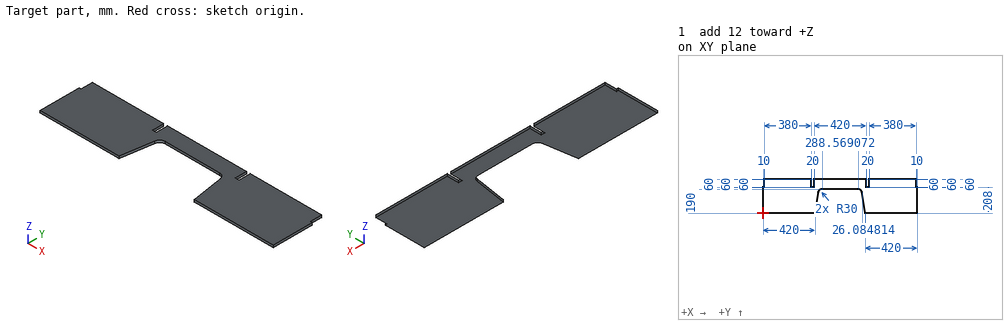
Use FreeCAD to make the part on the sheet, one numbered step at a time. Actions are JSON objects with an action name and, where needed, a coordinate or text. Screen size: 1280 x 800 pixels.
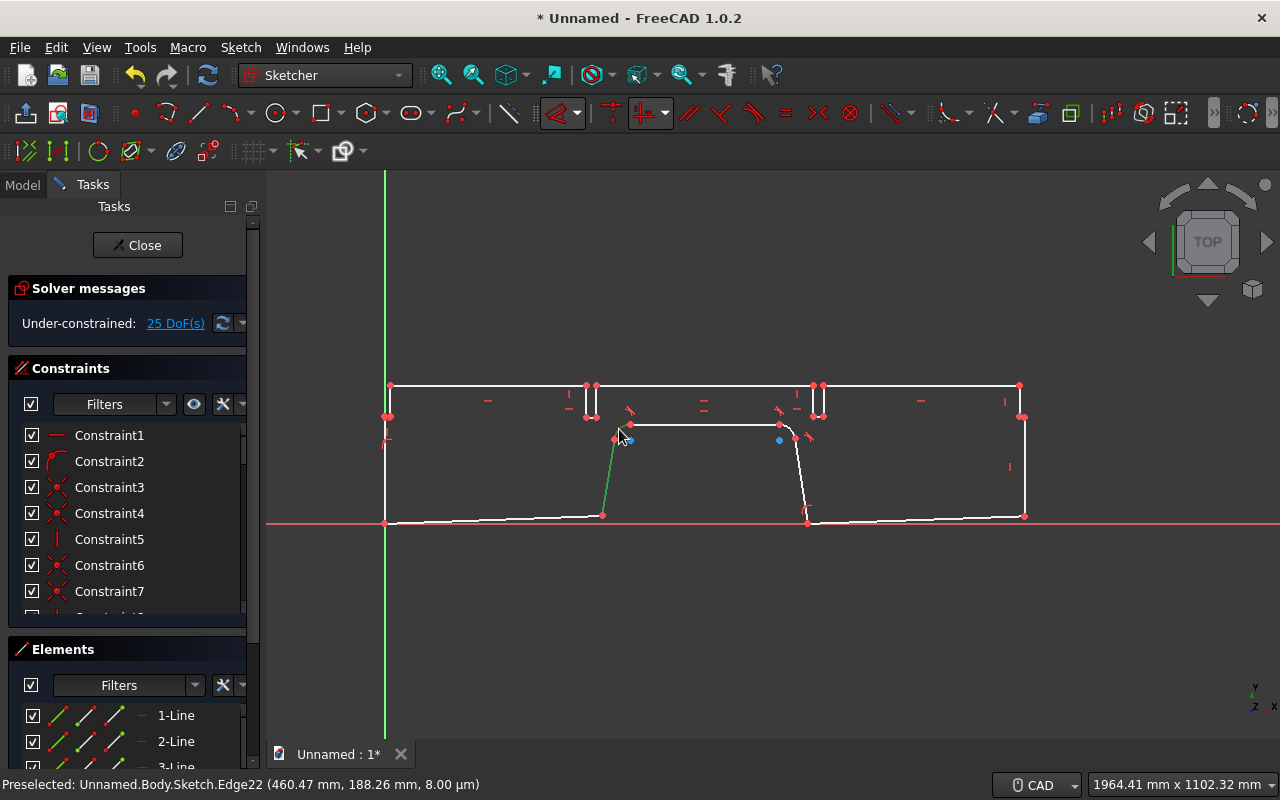
{"action": "key", "text": "t"}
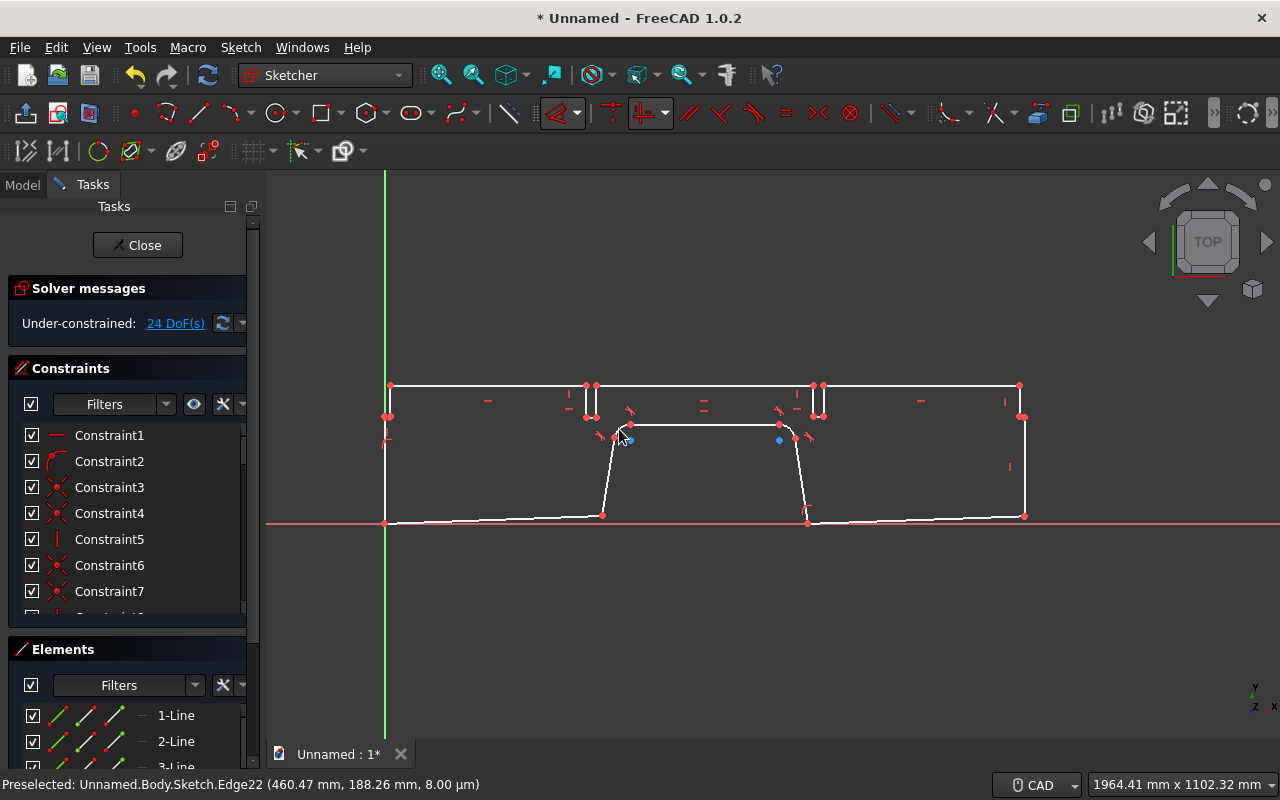
{"action": "left_click", "coordinate": [873, 522]}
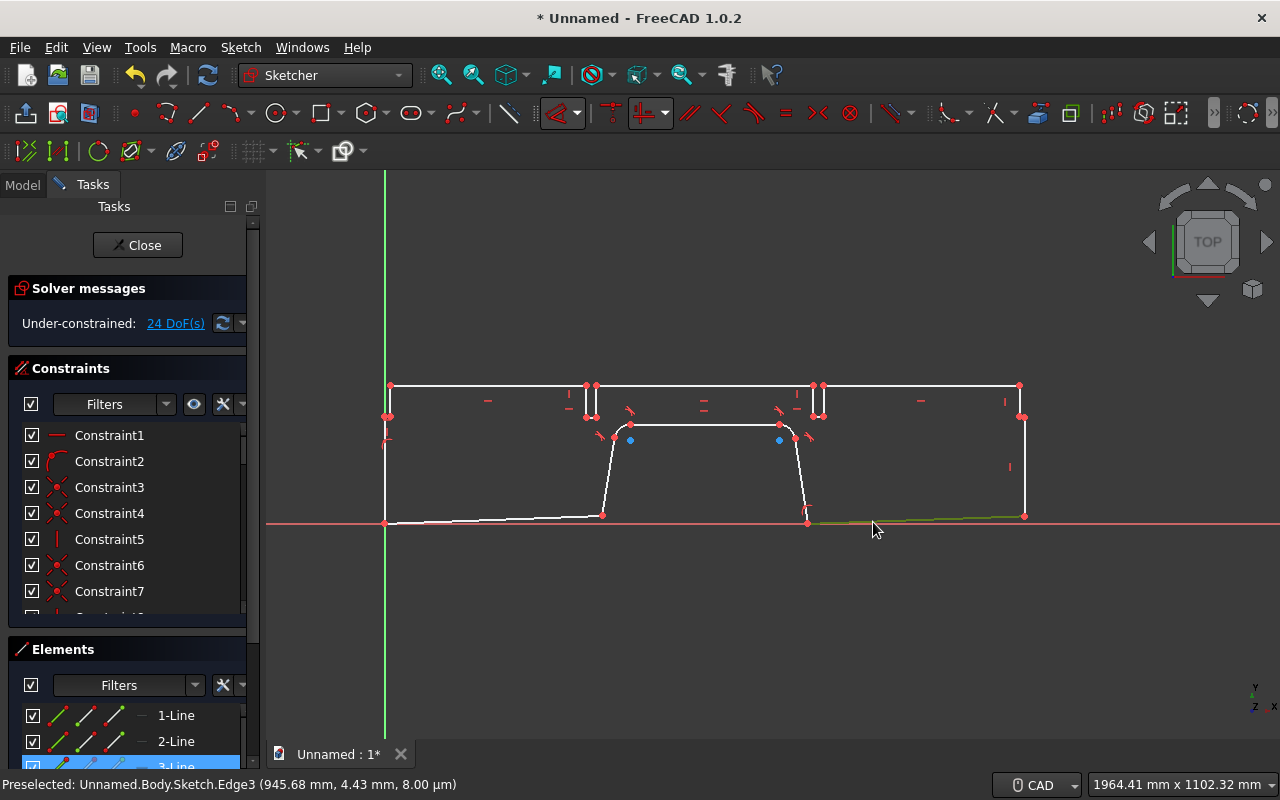
{"action": "key", "text": "h"}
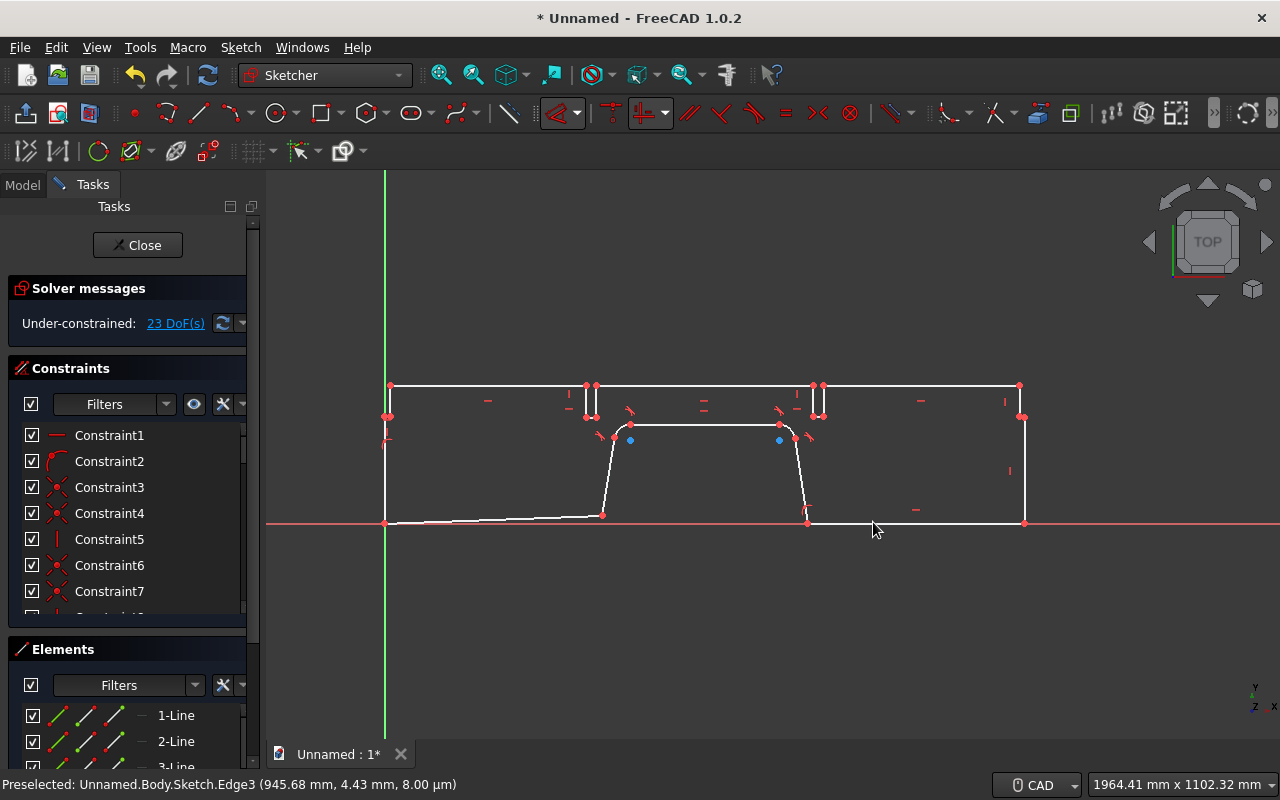
{"action": "scroll", "coordinate": [1022, 417], "scroll_direction": "up", "scroll_amount": 9}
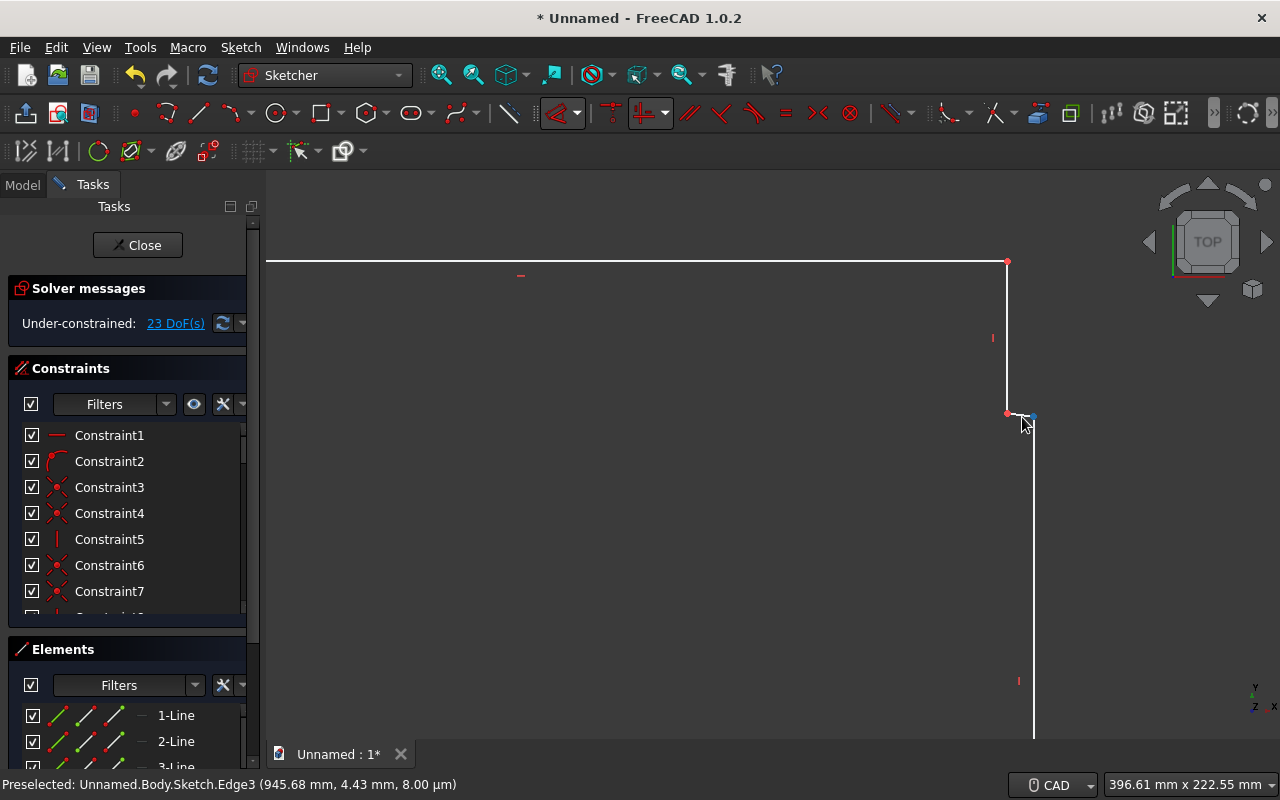
{"action": "left_click", "coordinate": [1020, 415]}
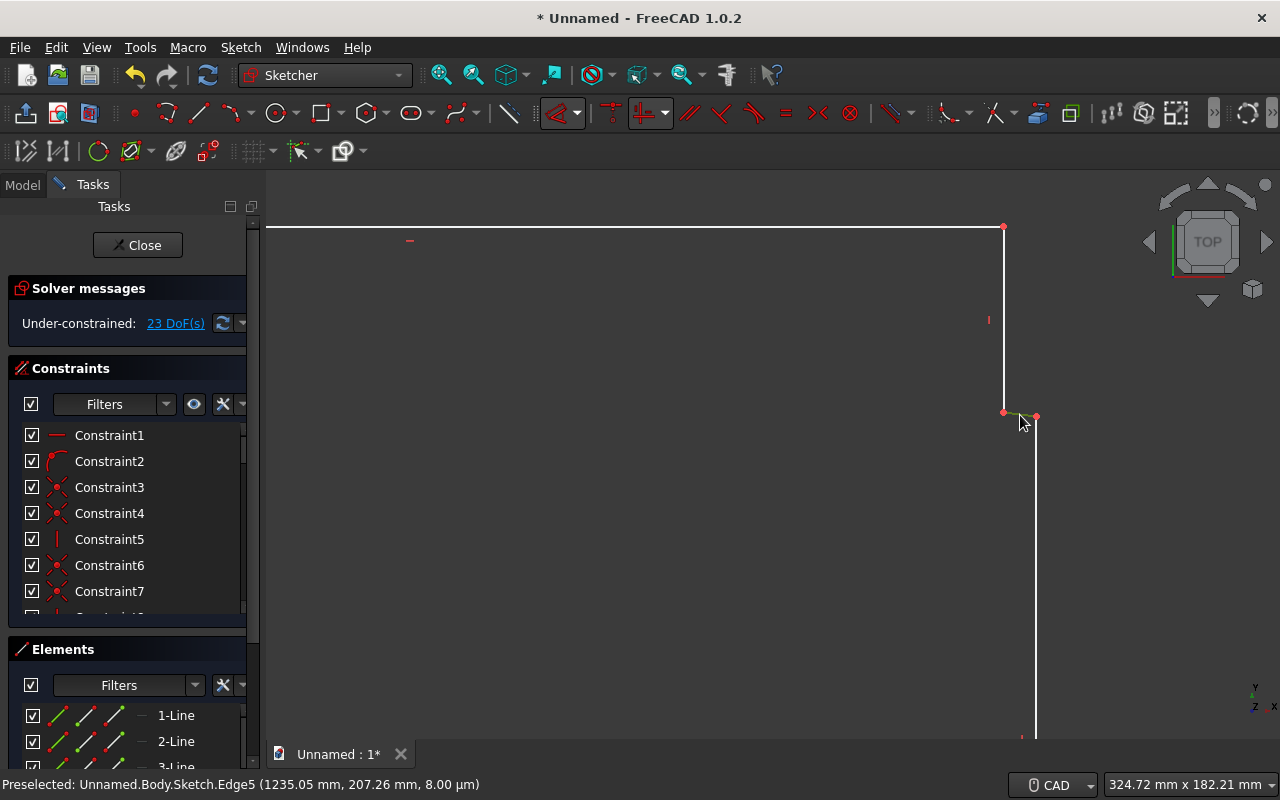
{"action": "key", "text": "h"}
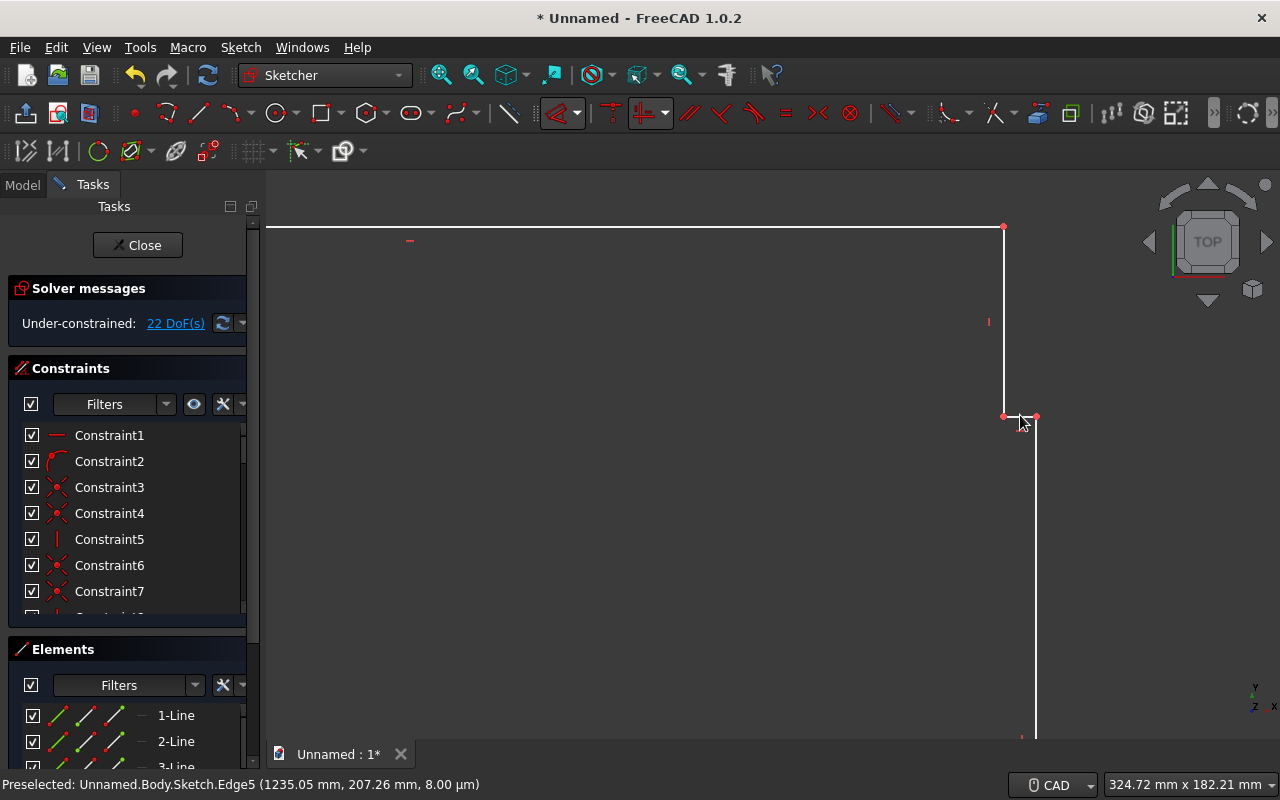
{"action": "scroll", "coordinate": [1022, 417], "scroll_direction": "down", "scroll_amount": 9}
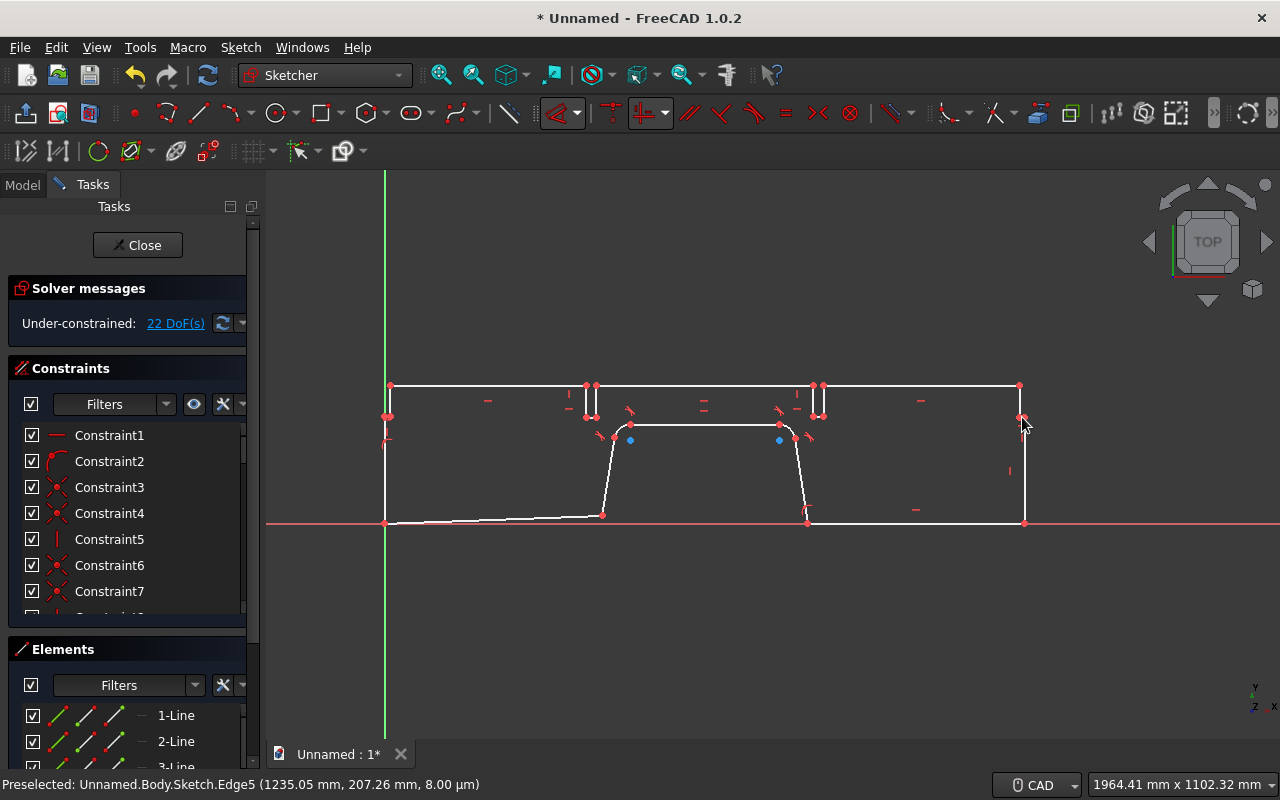
{"action": "scroll", "coordinate": [450, 522], "scroll_direction": "up", "scroll_amount": 9}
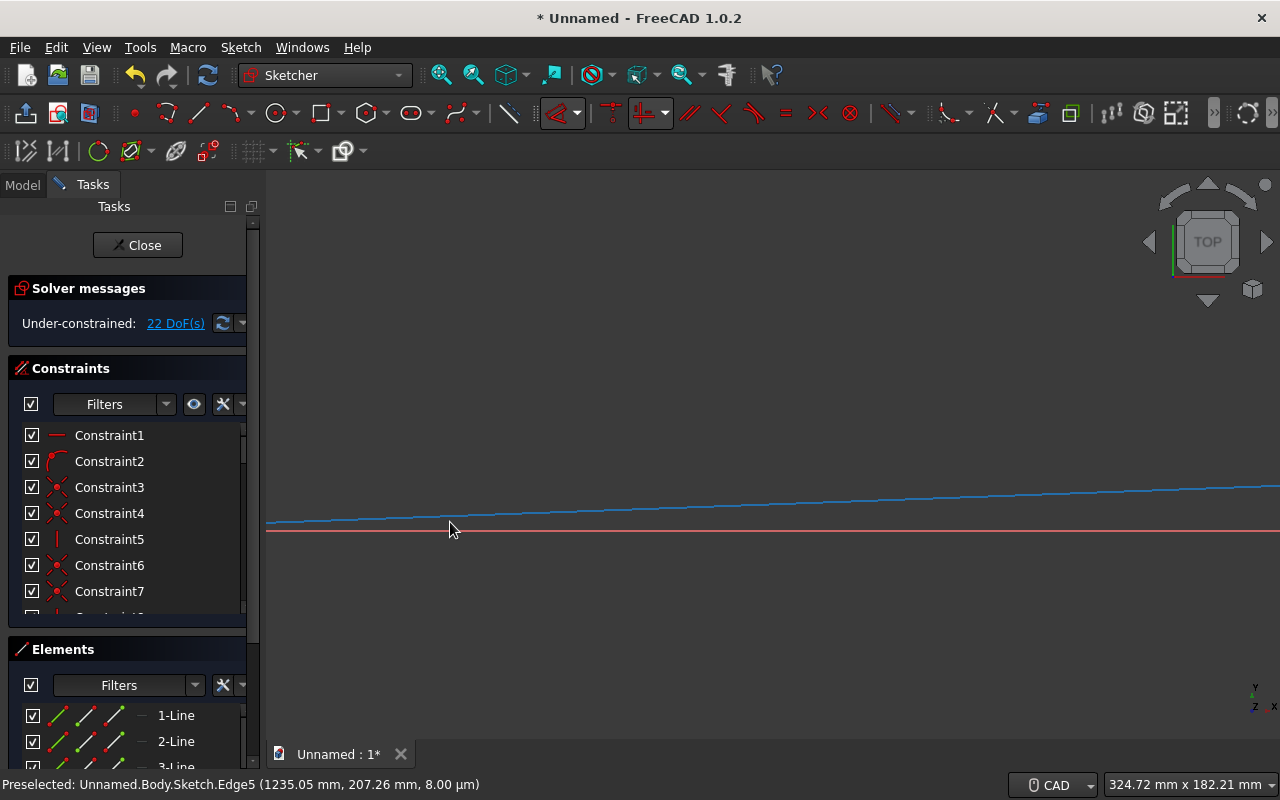
{"action": "left_click", "coordinate": [449, 516]}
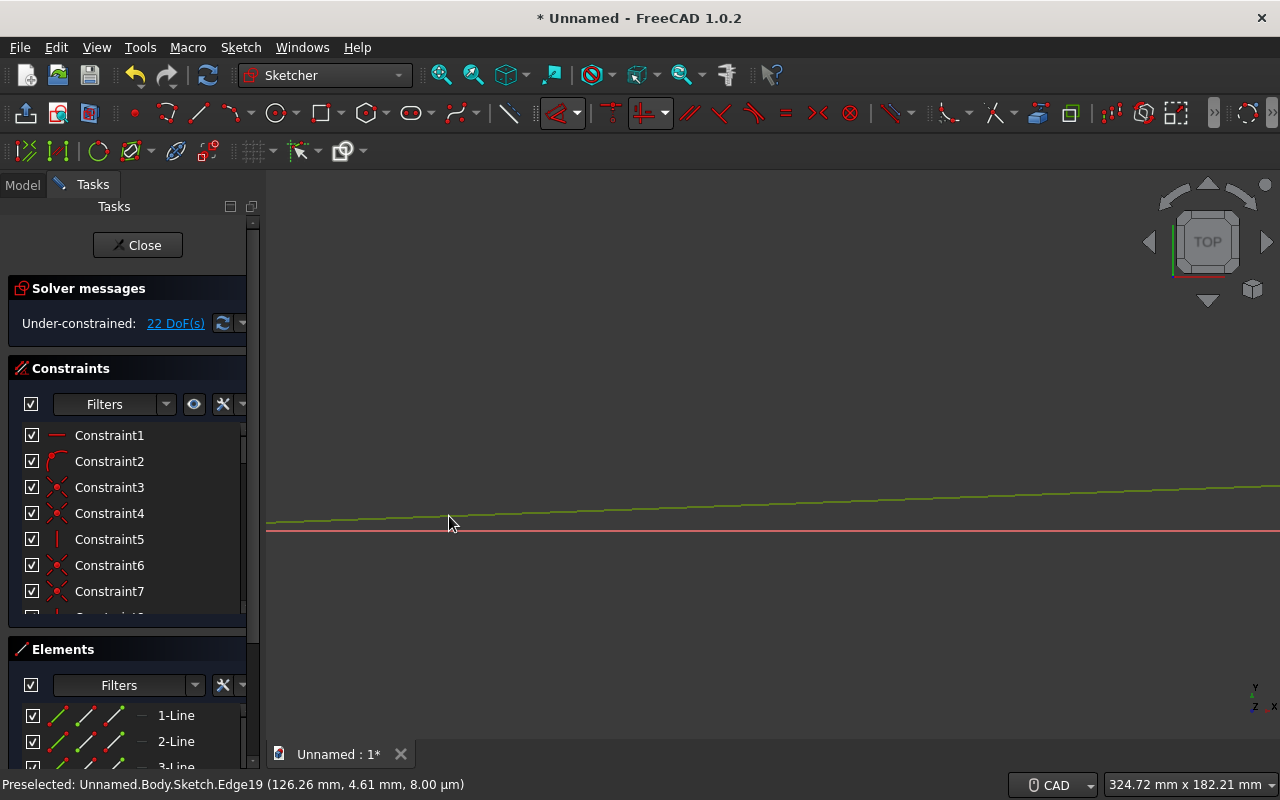
{"action": "key", "text": "h"}